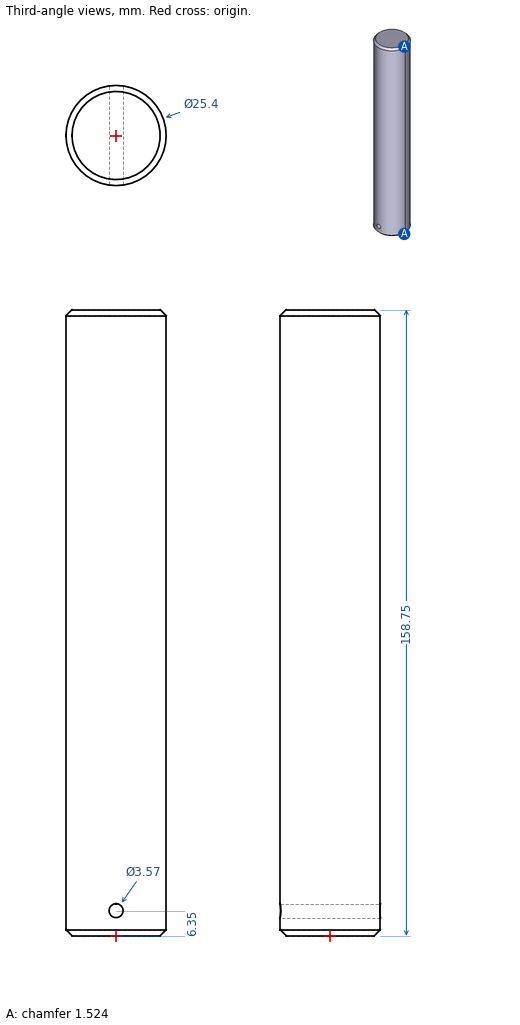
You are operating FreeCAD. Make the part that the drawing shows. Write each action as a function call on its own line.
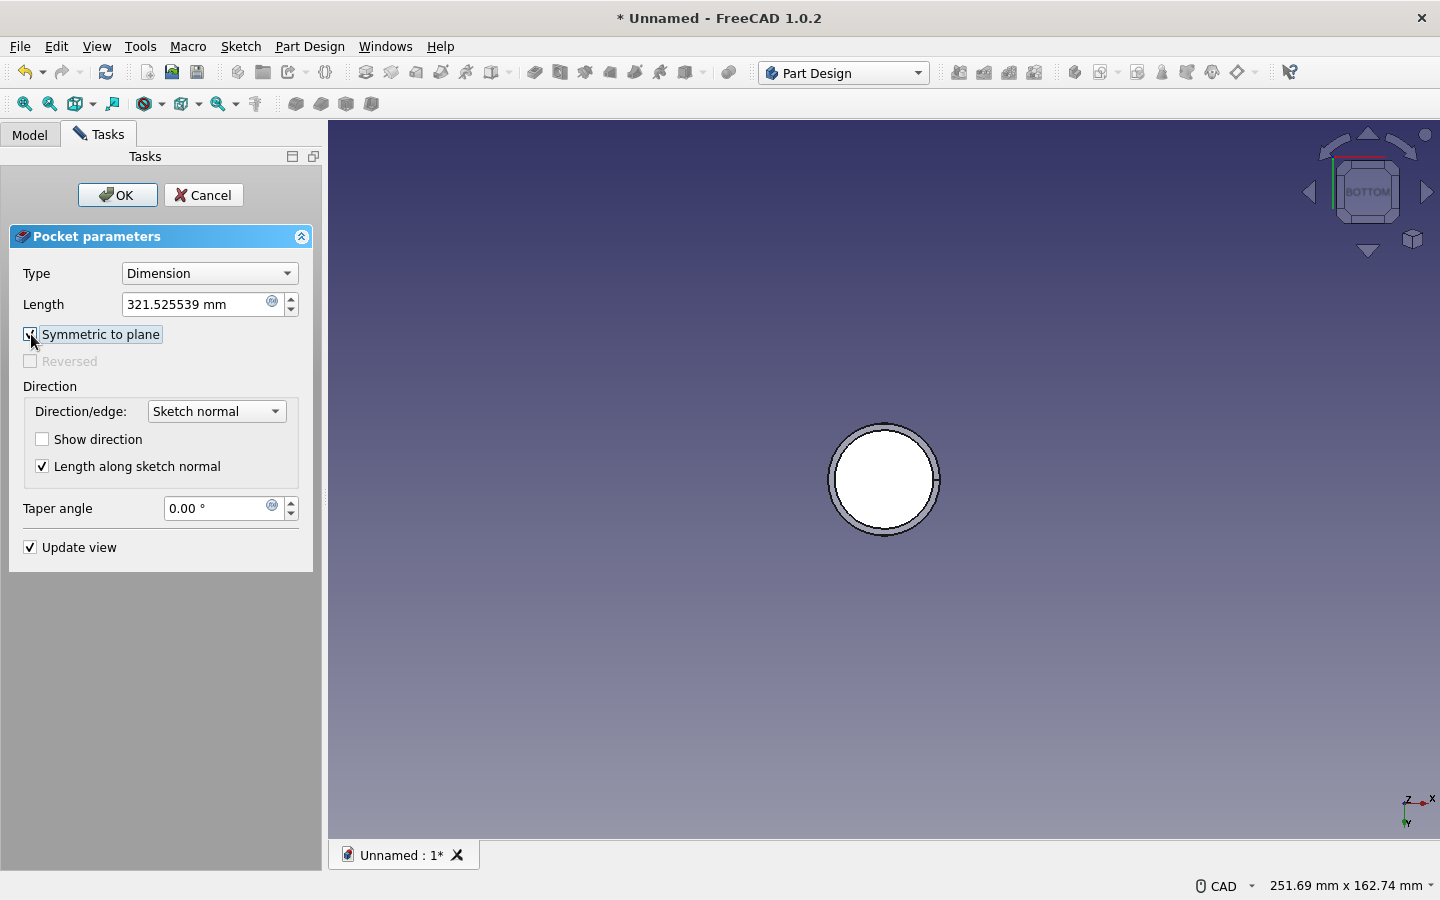
click(118, 195)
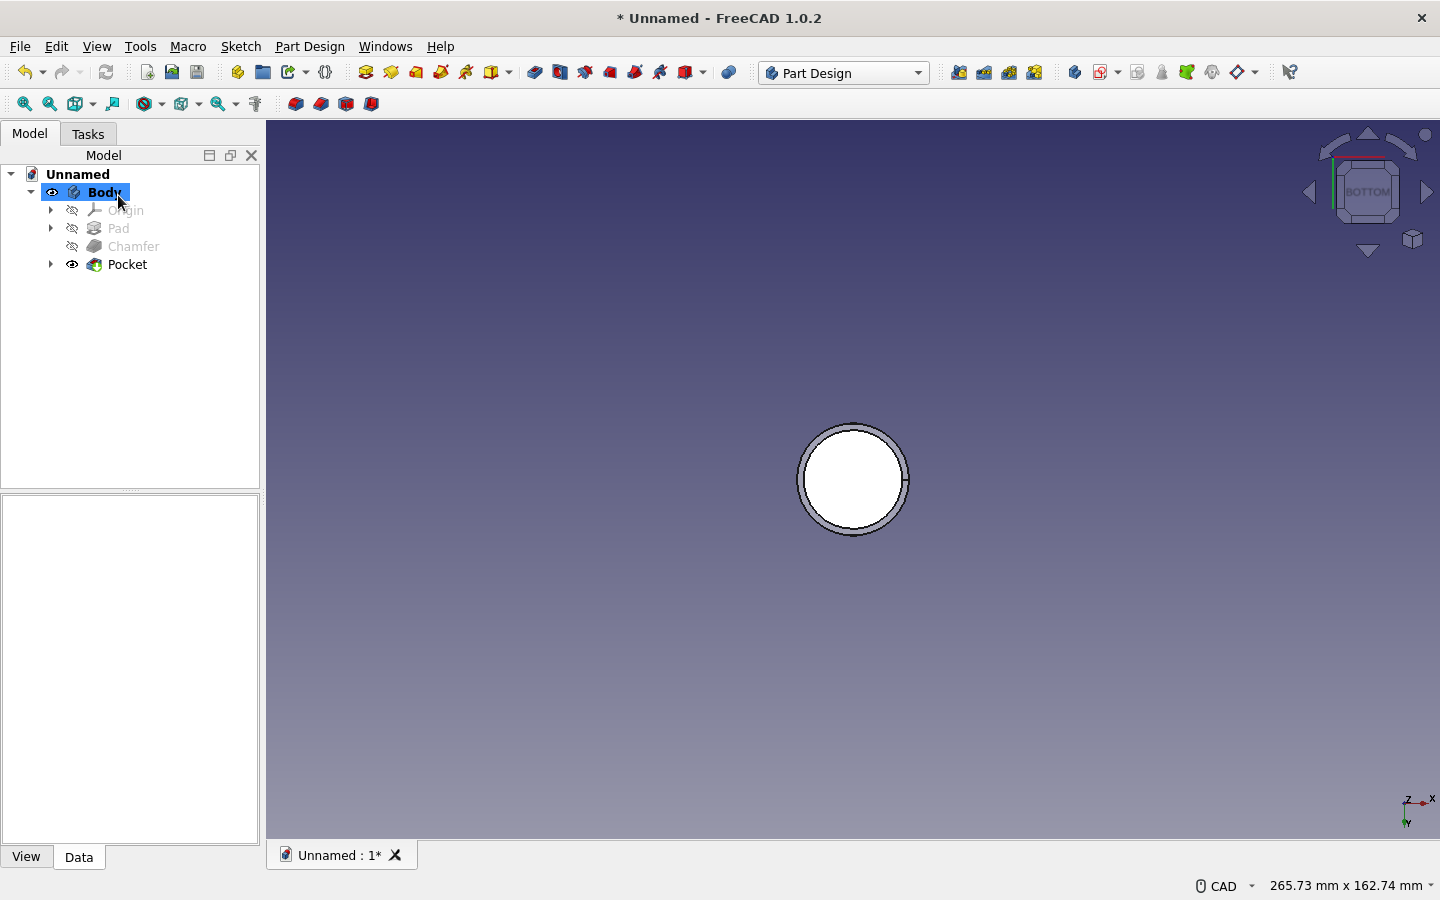
key(0)